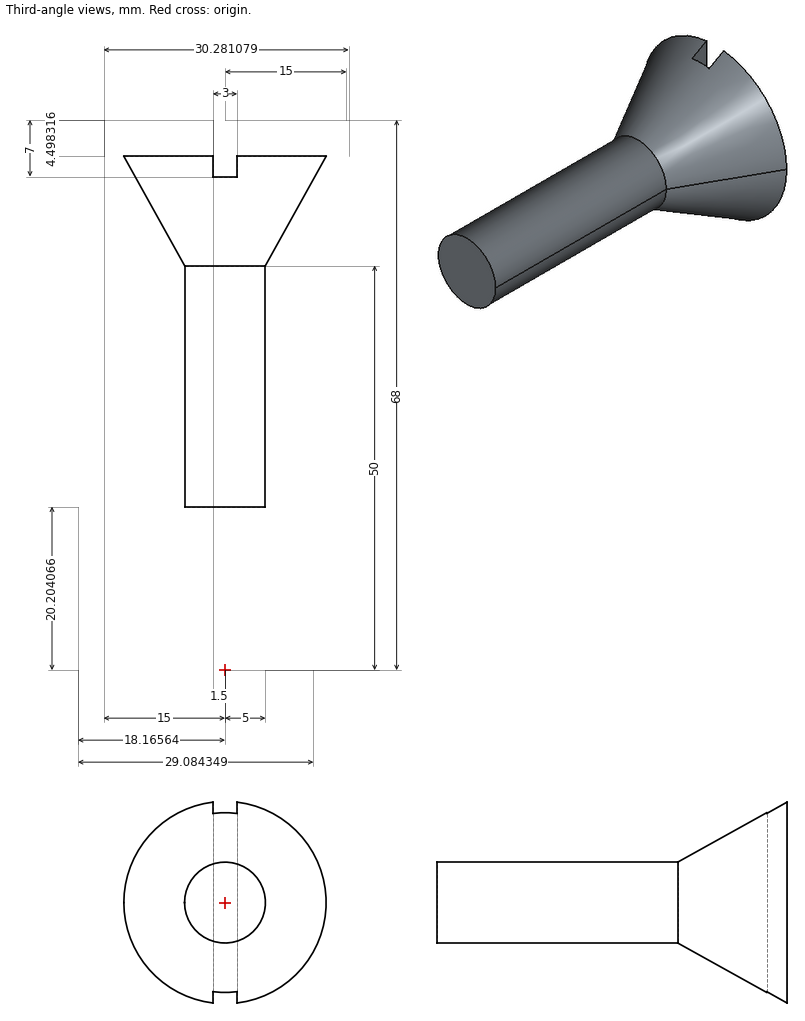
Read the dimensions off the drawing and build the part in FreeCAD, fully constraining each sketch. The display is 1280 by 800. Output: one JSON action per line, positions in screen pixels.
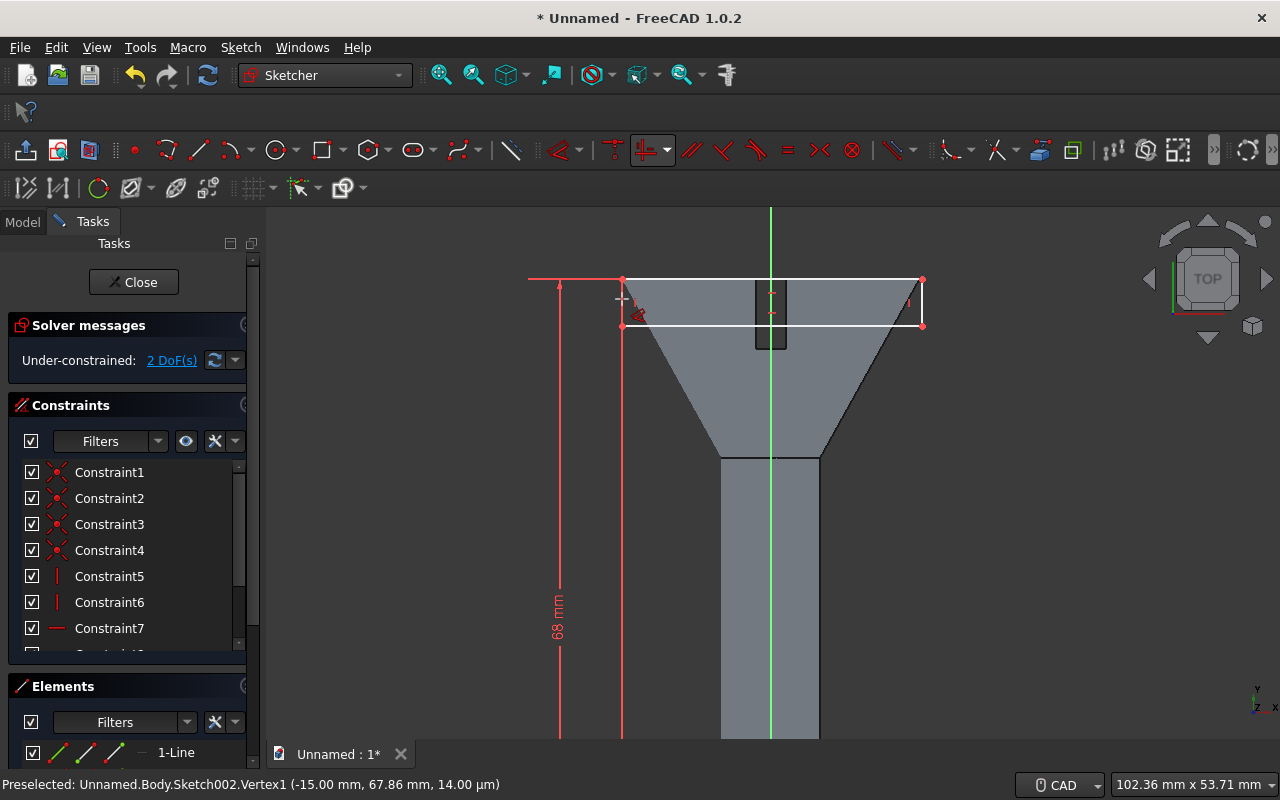
{"action": "left_click", "coordinate": [622, 298]}
{"action": "left_click", "coordinate": [588, 303]}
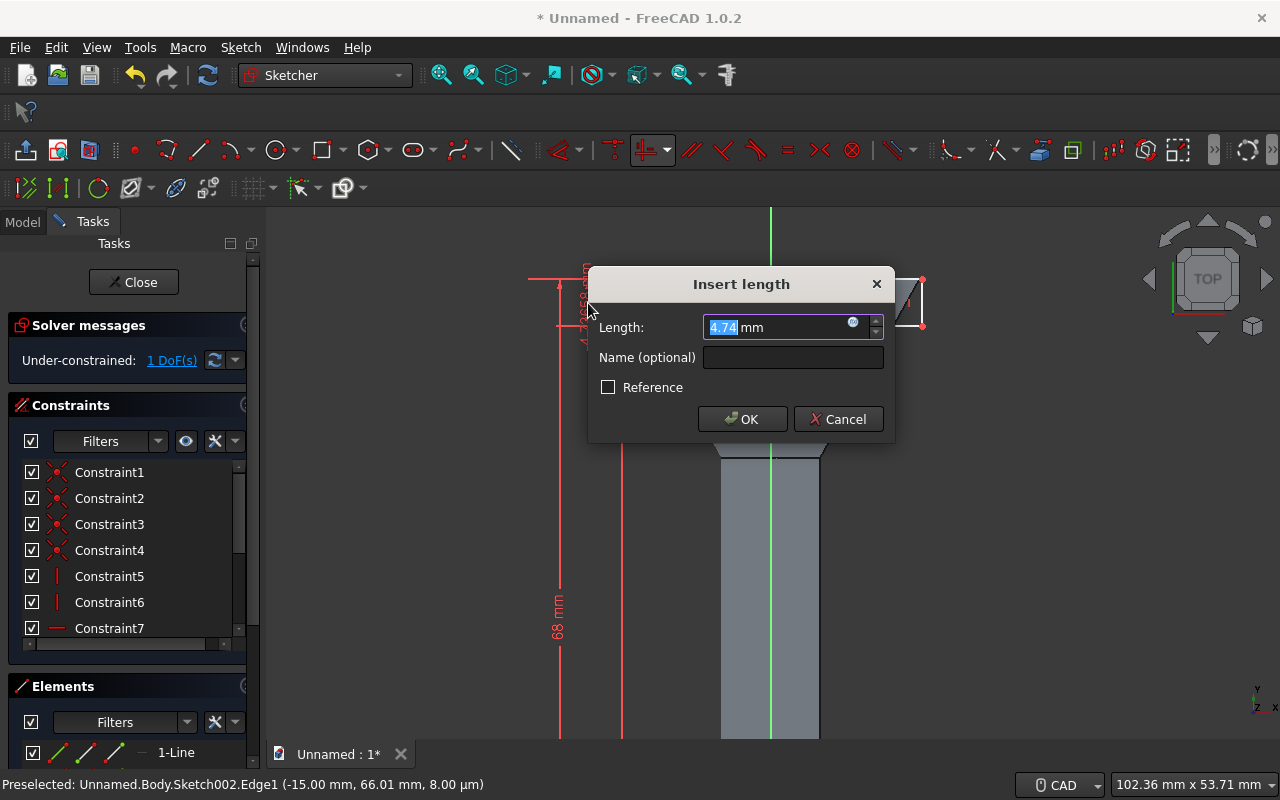
{"action": "type", "text": "4.498316"}
{"action": "key", "text": "Return"}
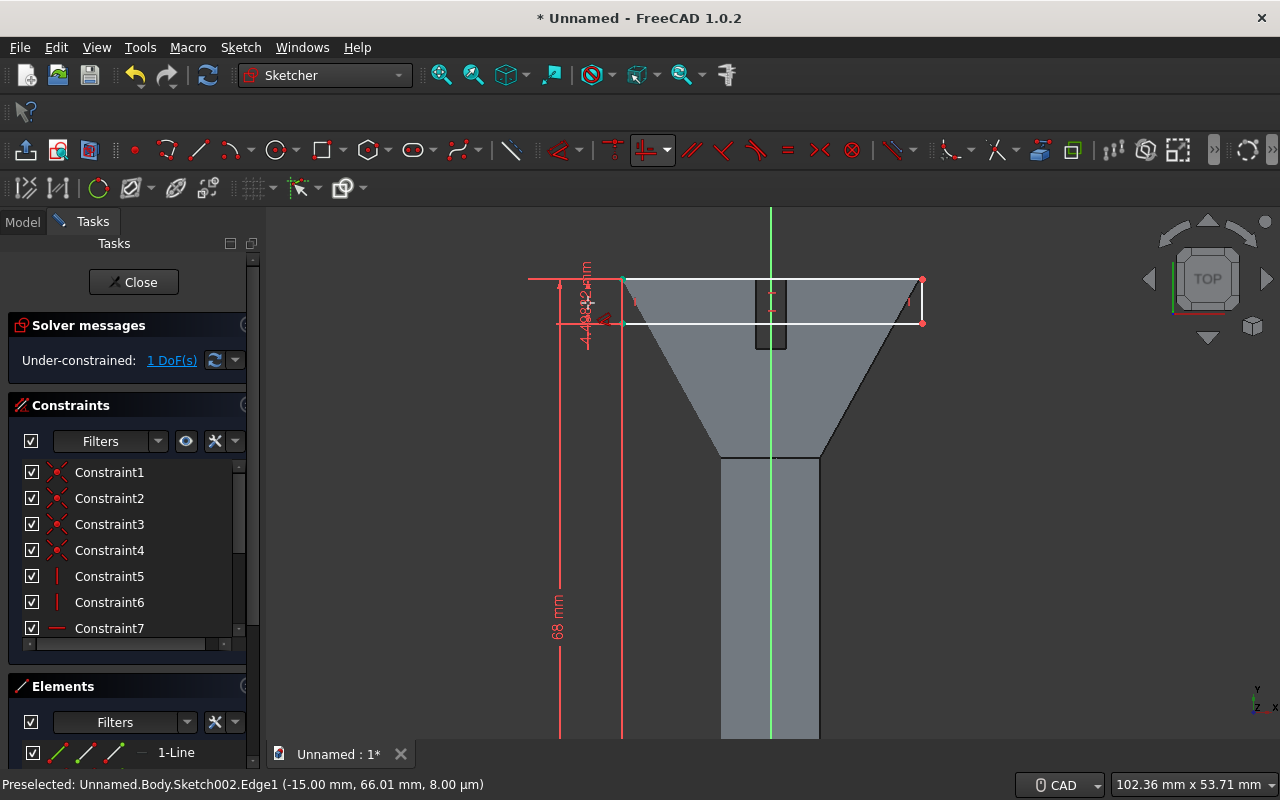
{"action": "left_click", "coordinate": [712, 324]}
{"action": "left_click", "coordinate": [703, 358]}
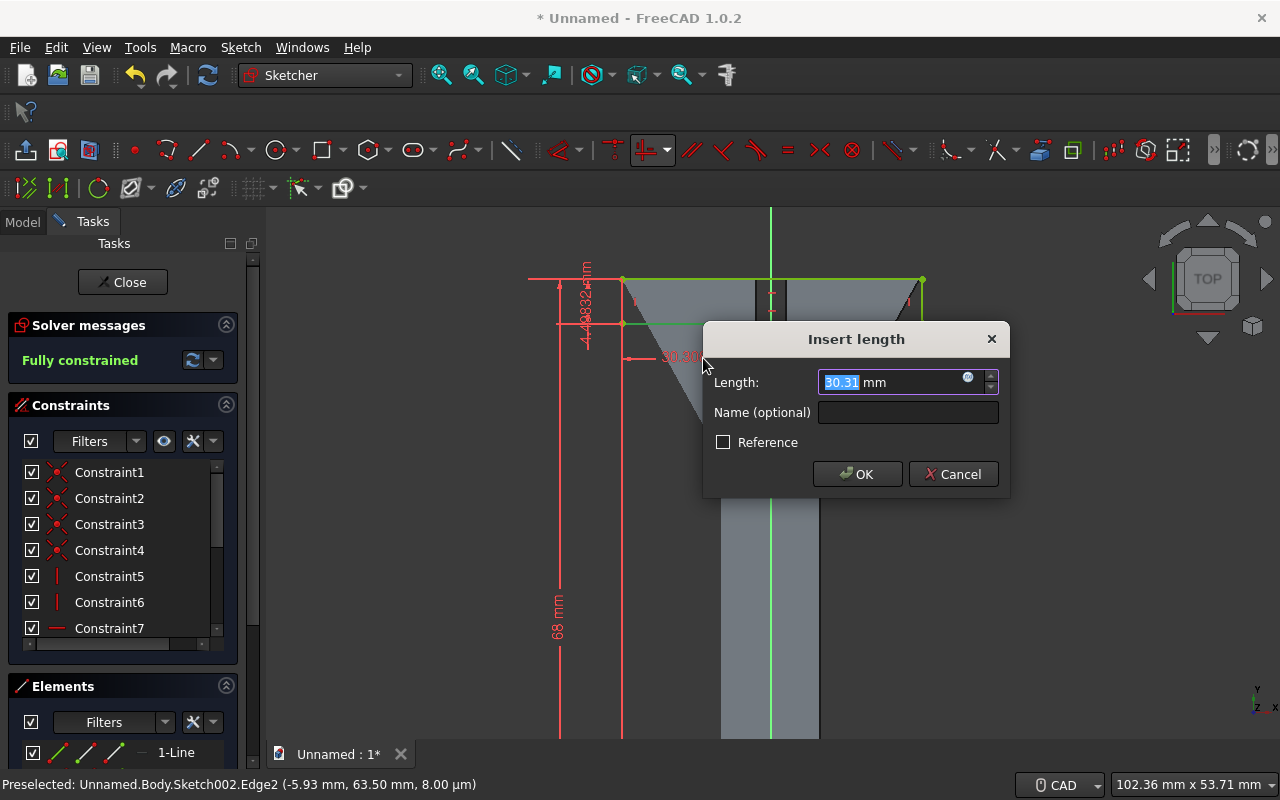
{"action": "type", "text": "30.281079"}
{"action": "key", "text": "Return"}
{"action": "key", "text": "Escape"}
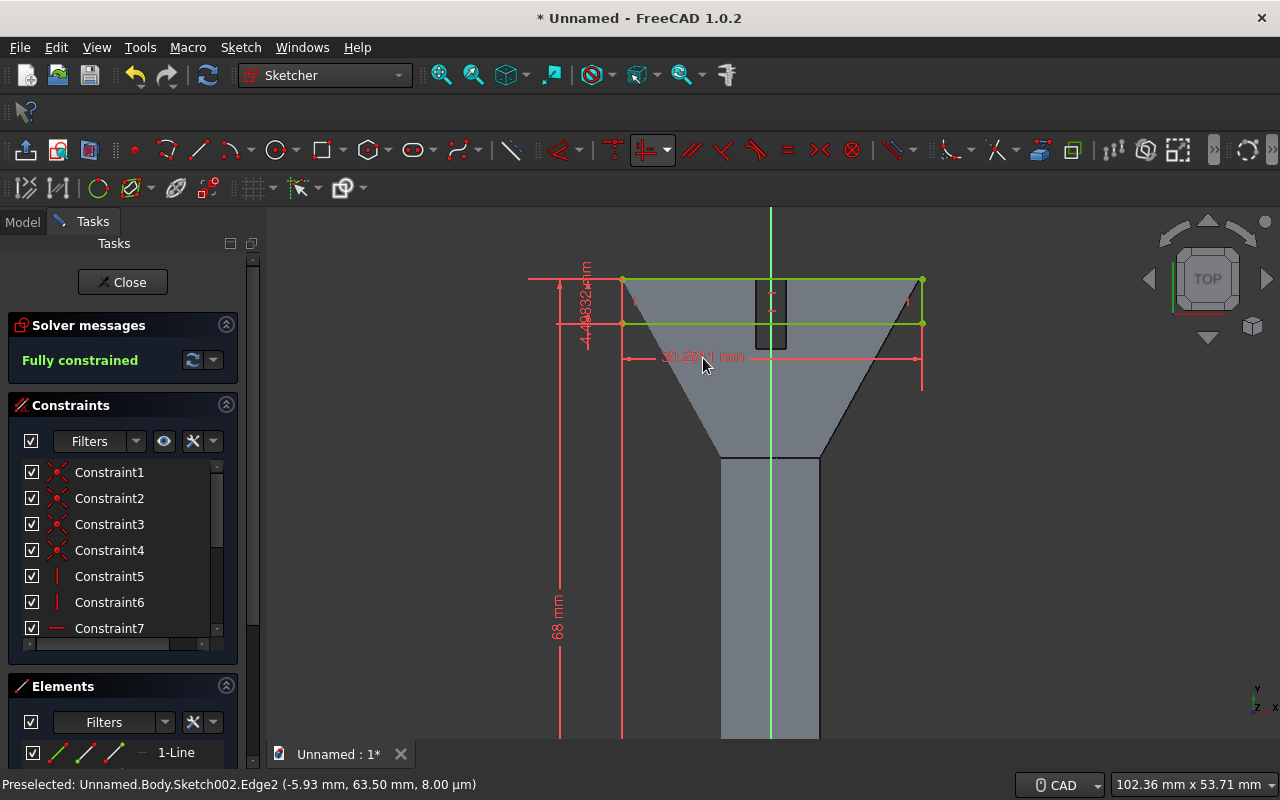
{"action": "left_click", "coordinate": [123, 282]}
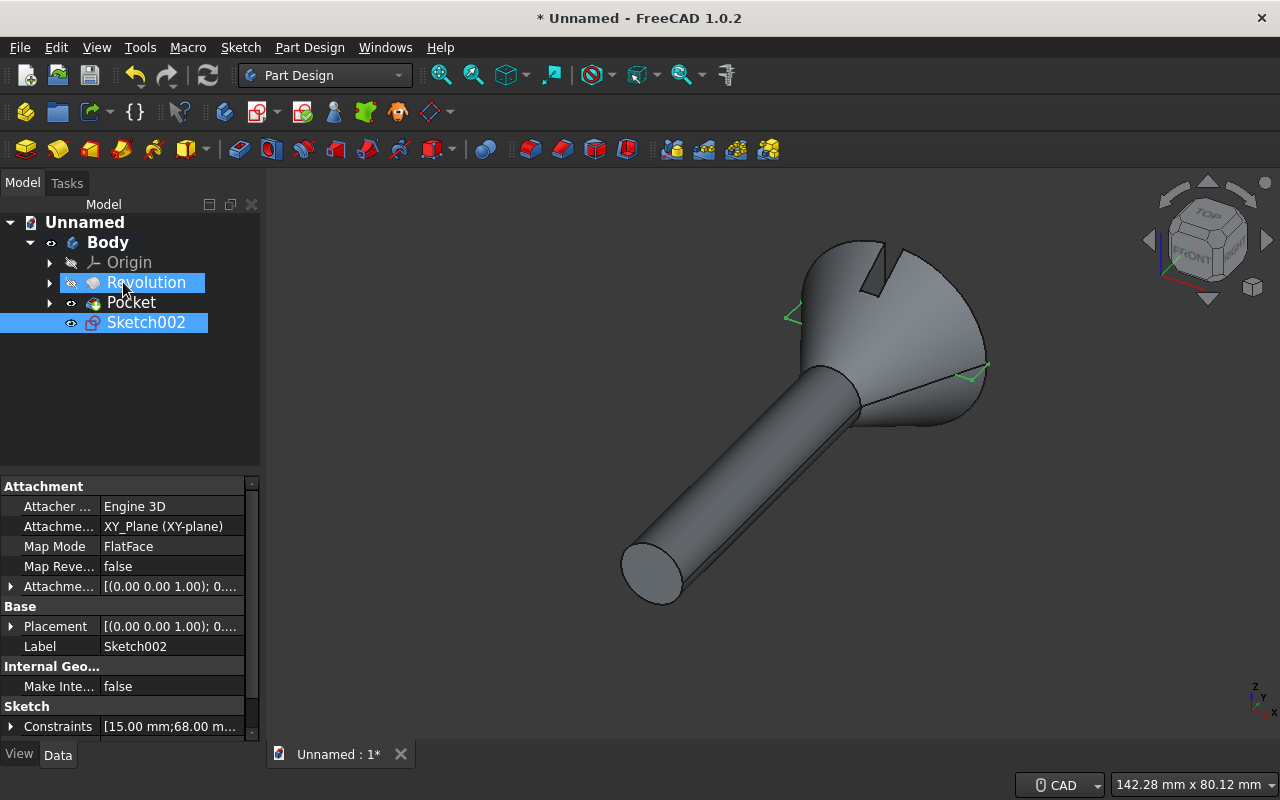
{"action": "left_click", "coordinate": [240, 150]}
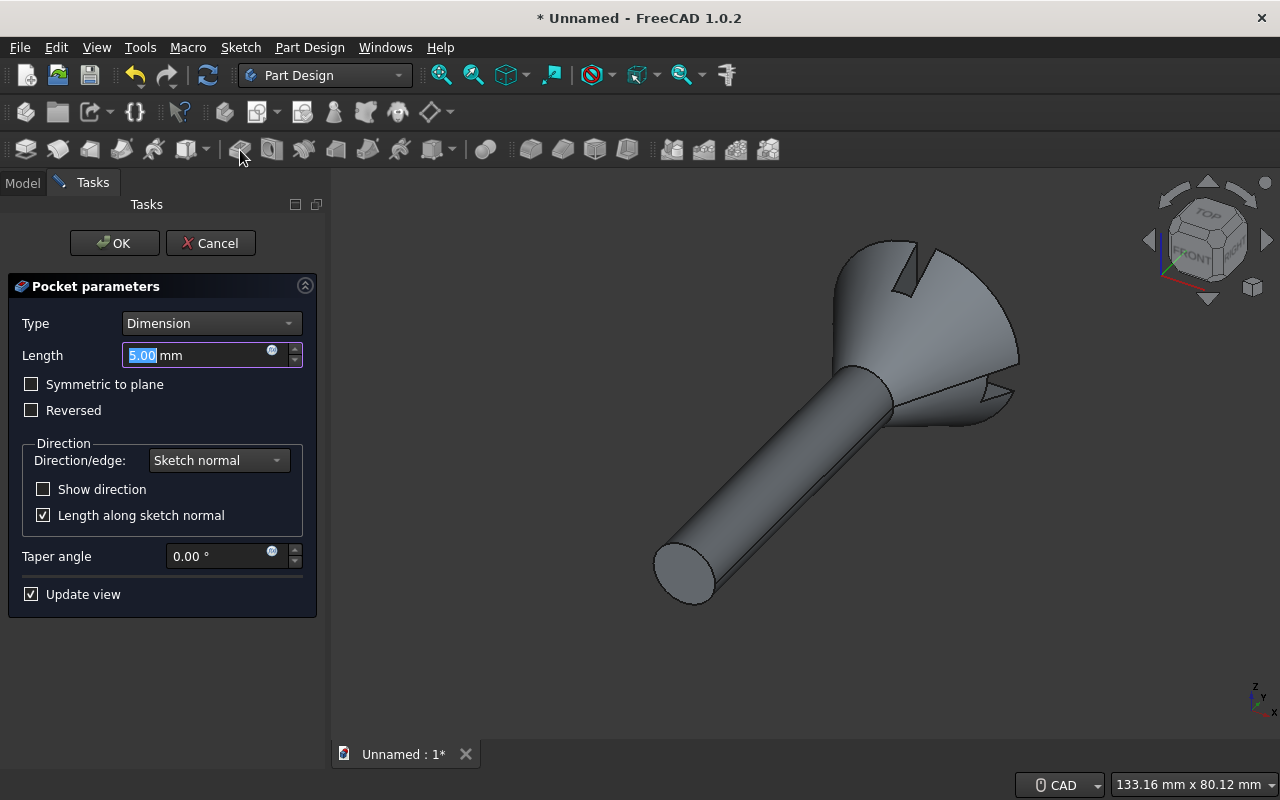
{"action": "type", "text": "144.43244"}
{"action": "key", "text": "Tab"}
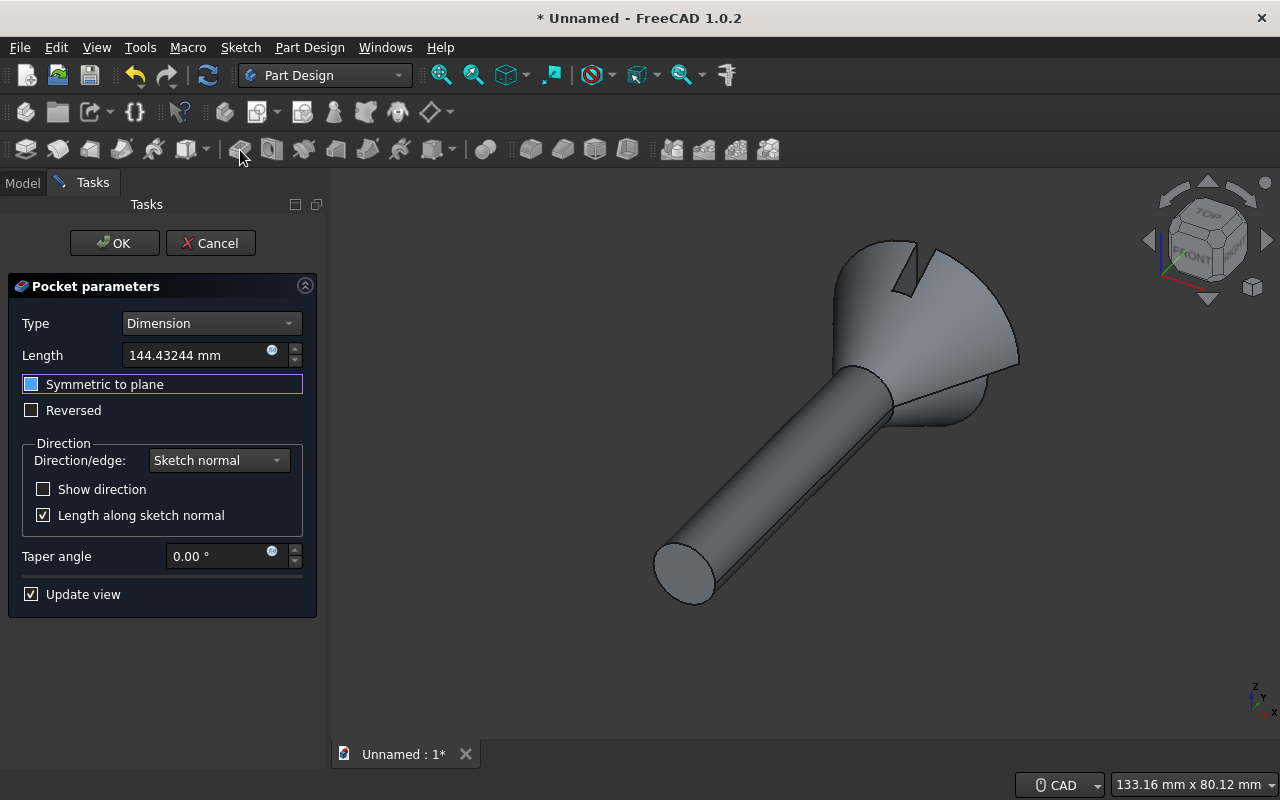
{"action": "left_click", "coordinate": [30, 384]}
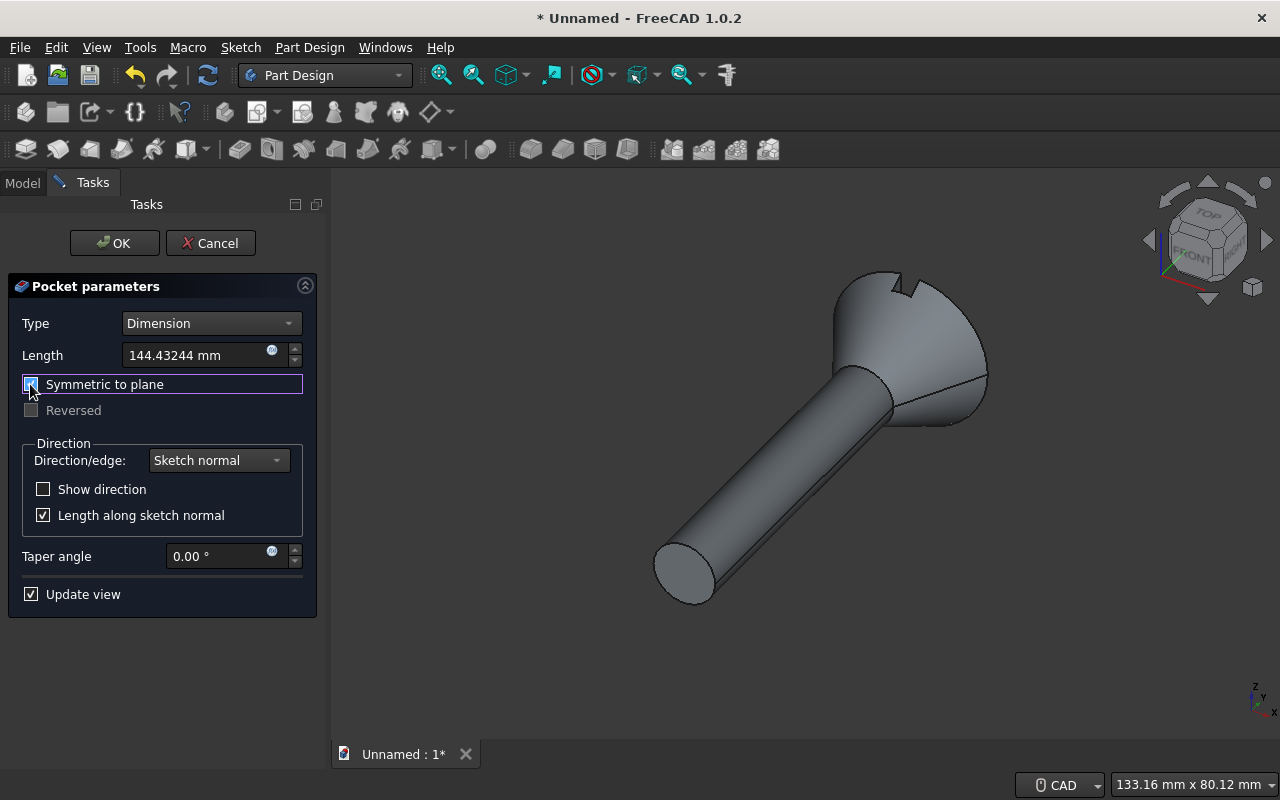
{"action": "left_click", "coordinate": [115, 243]}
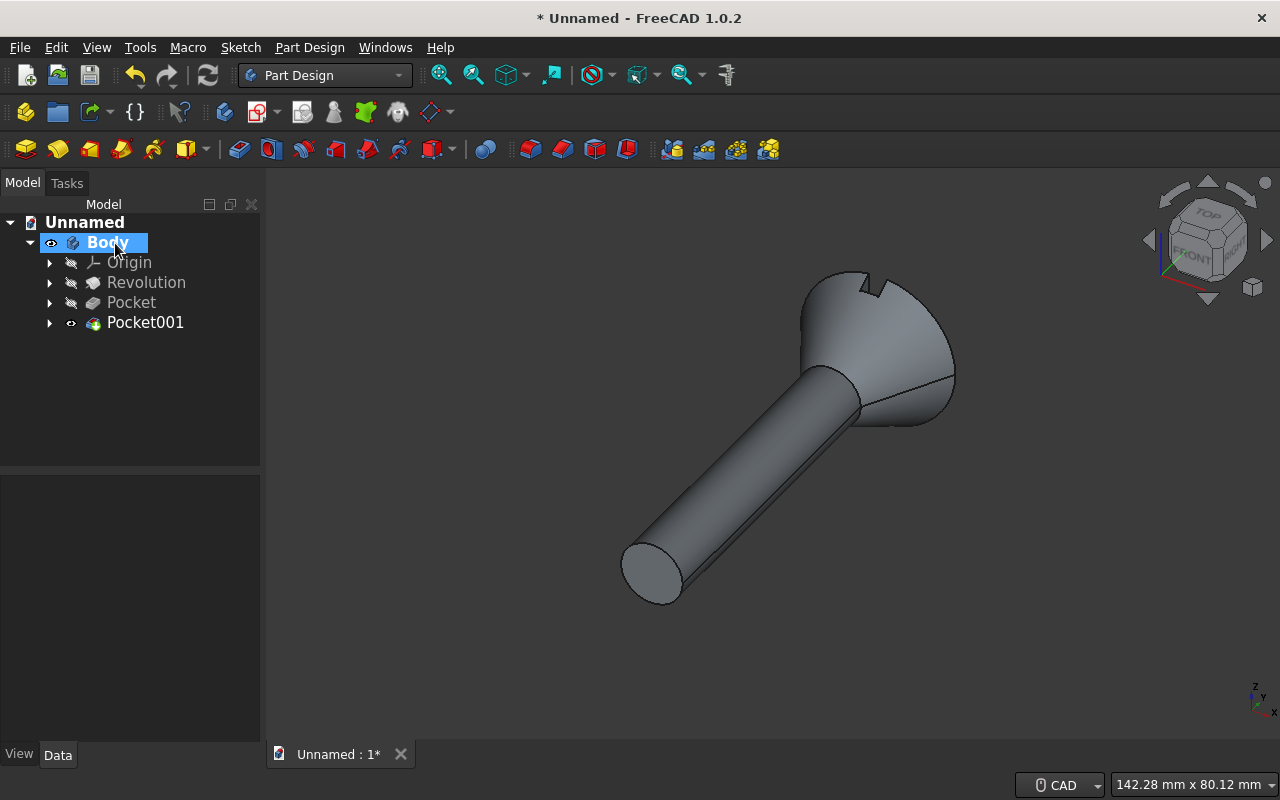
{"action": "left_click", "coordinate": [258, 112]}